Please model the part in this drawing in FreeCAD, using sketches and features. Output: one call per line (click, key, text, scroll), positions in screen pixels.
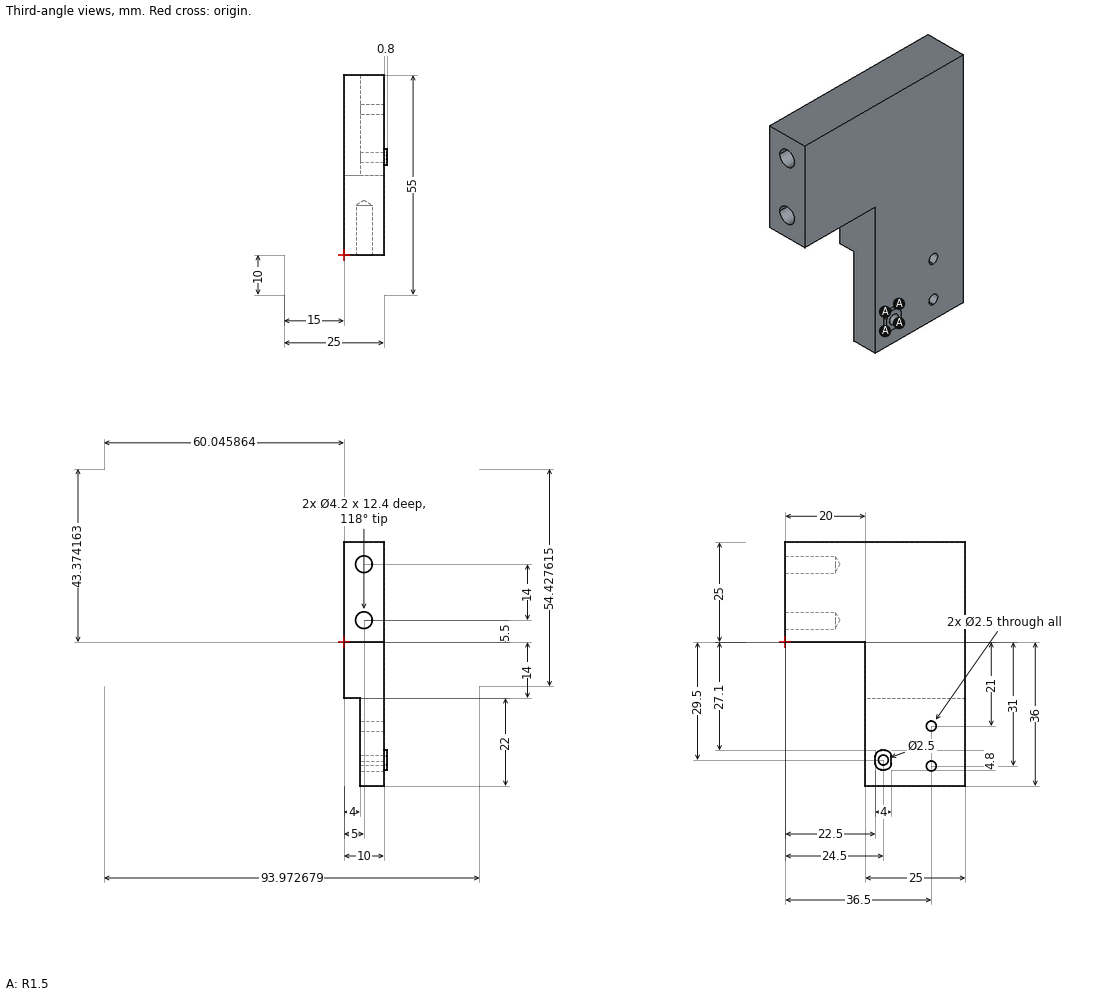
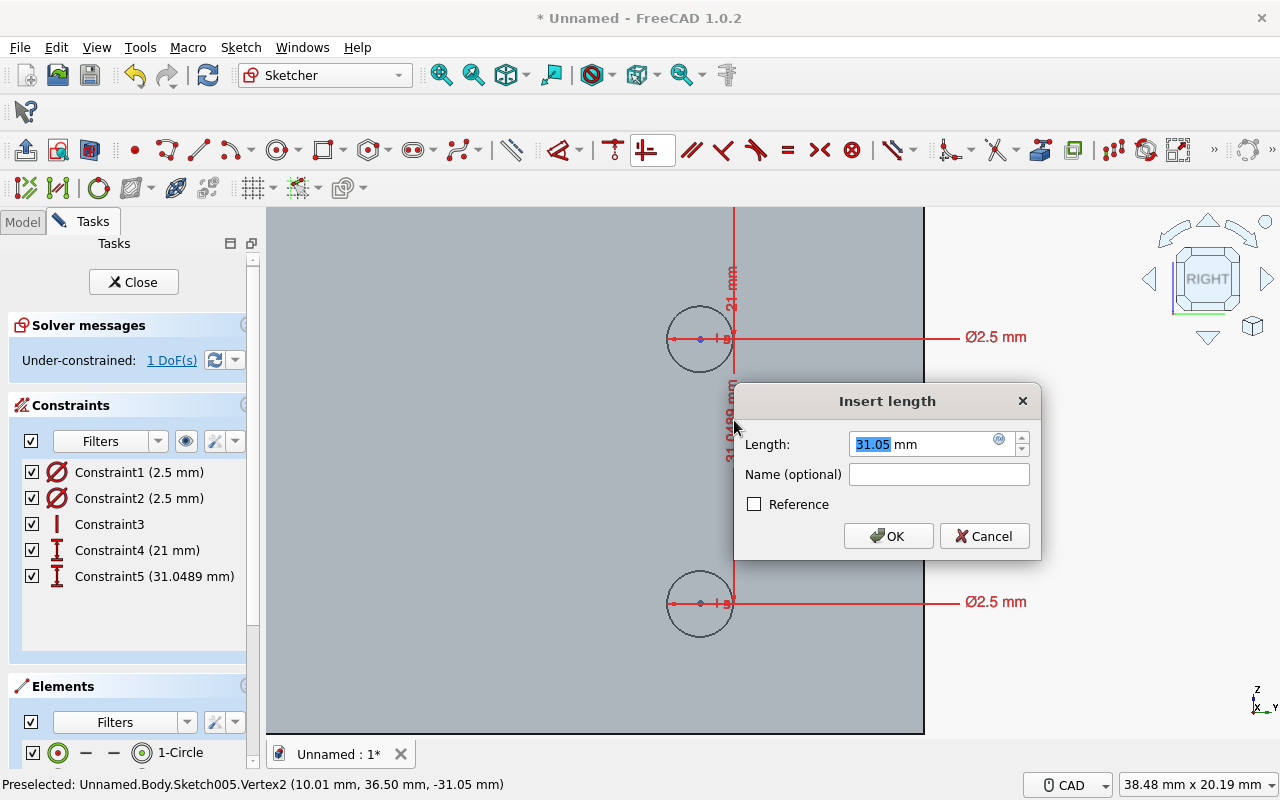
text(31)
key(Return)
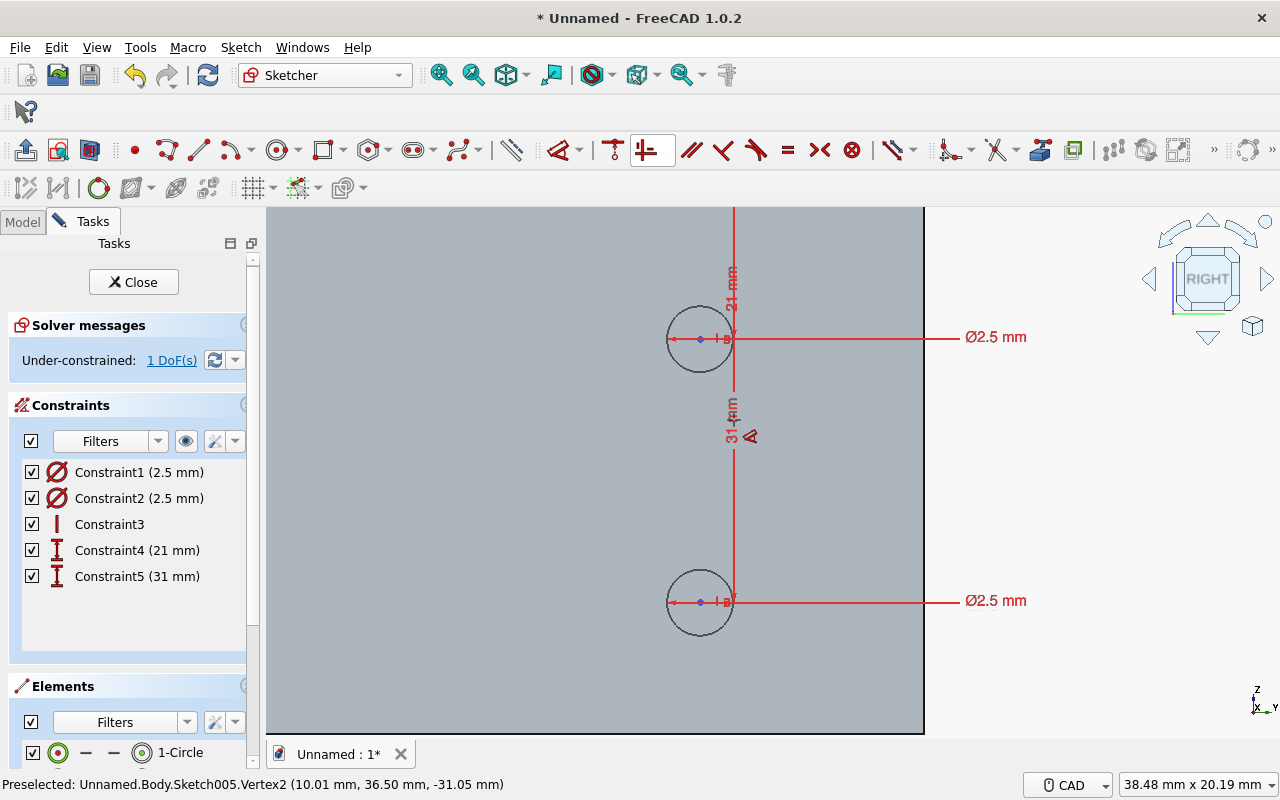
click(700, 339)
click(497, 373)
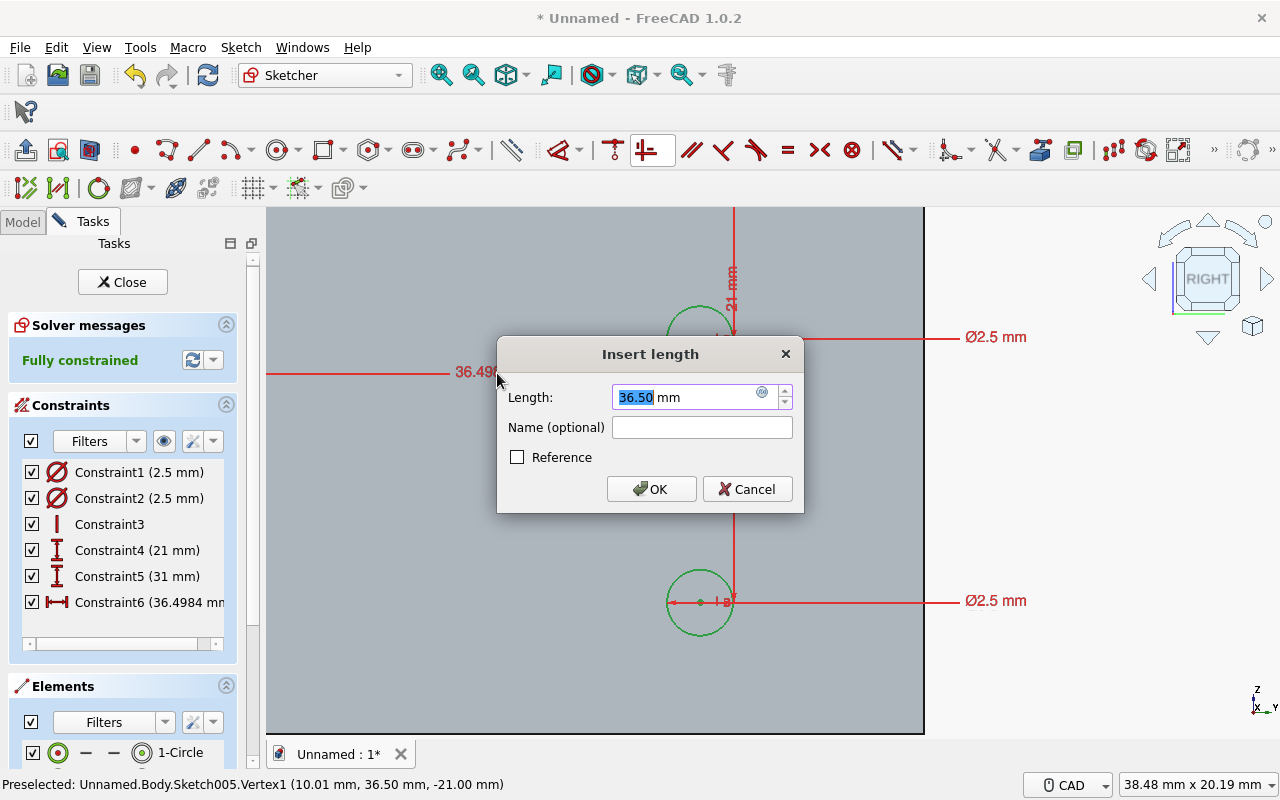
text(36.5)
key(Return)
key(Escape)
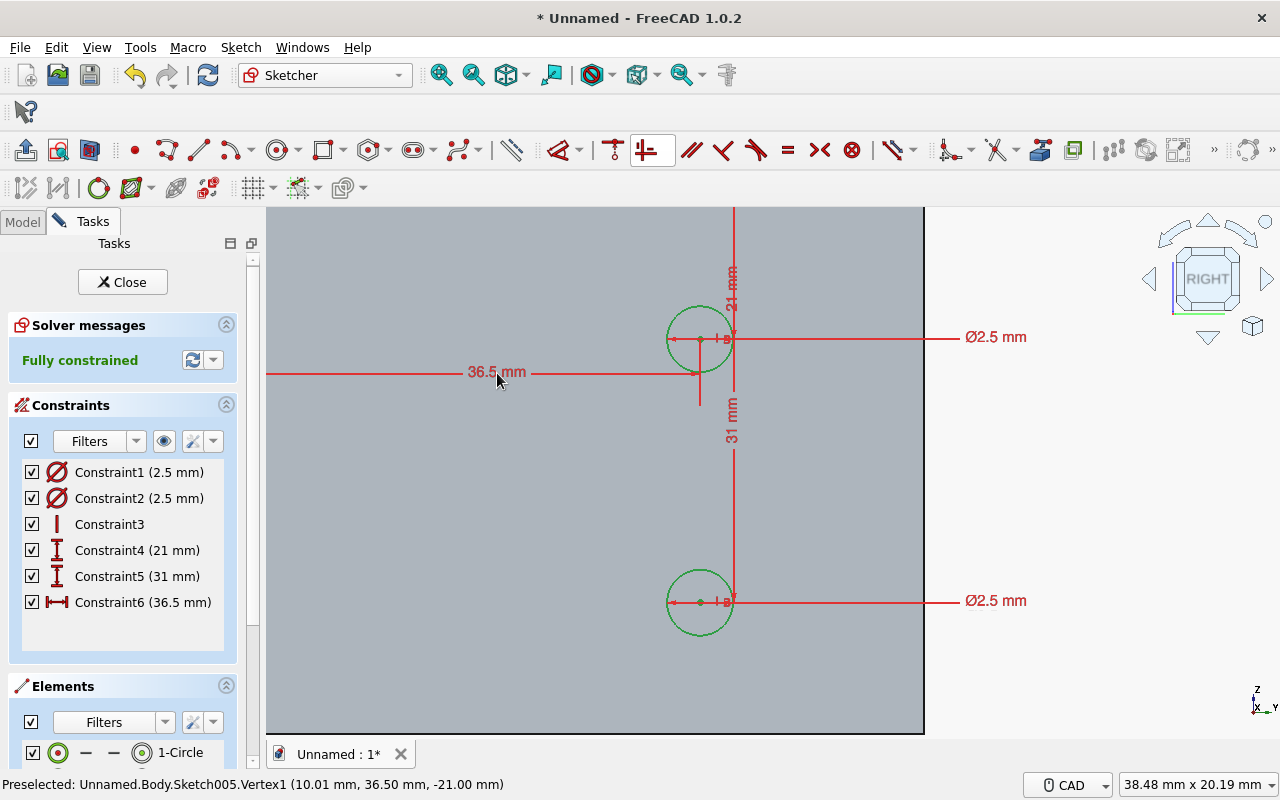
click(123, 282)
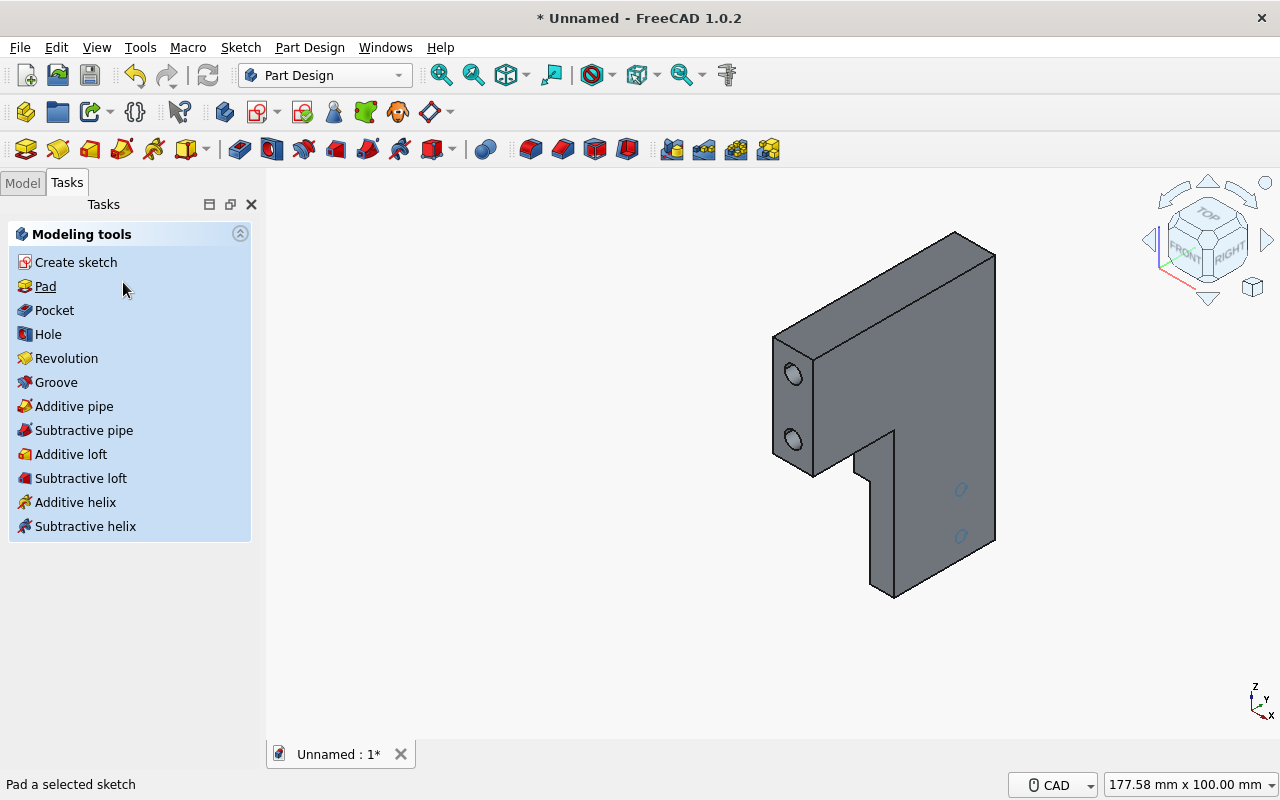
click(272, 150)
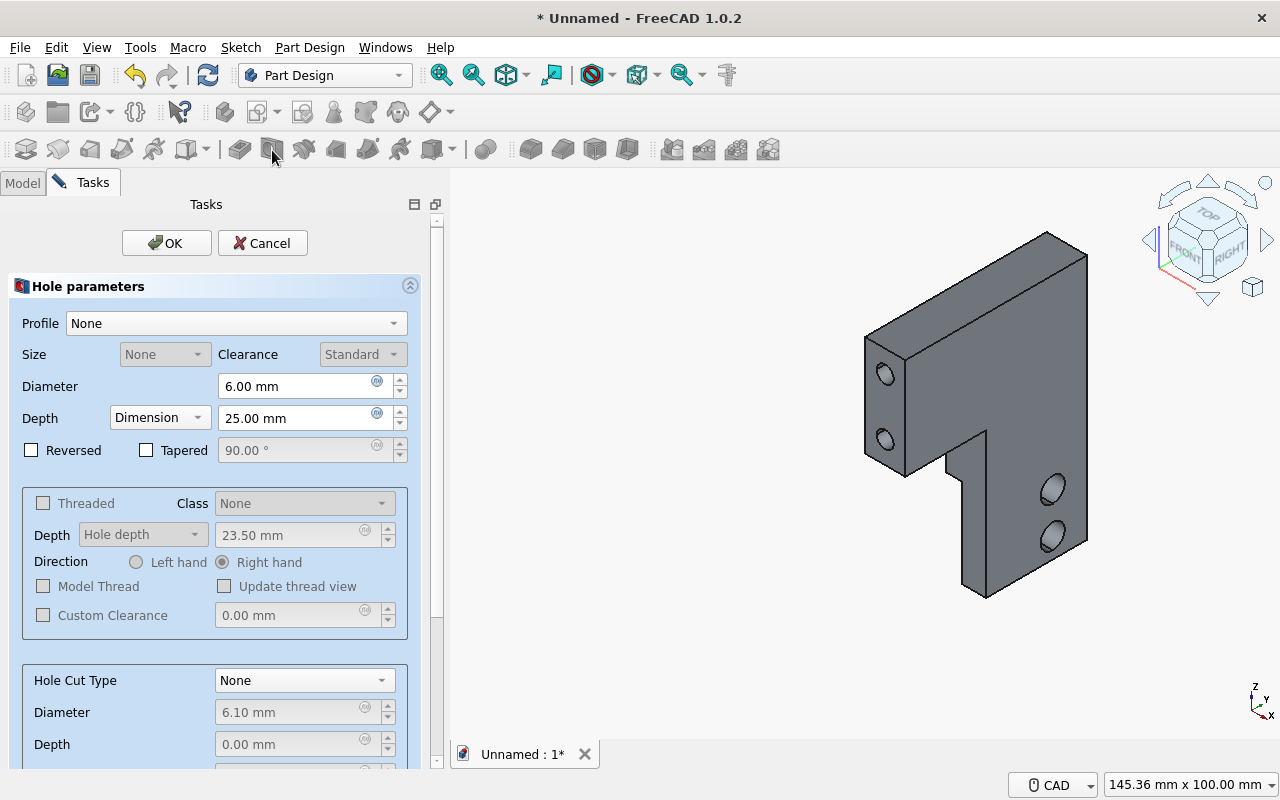
triple_click(305, 386)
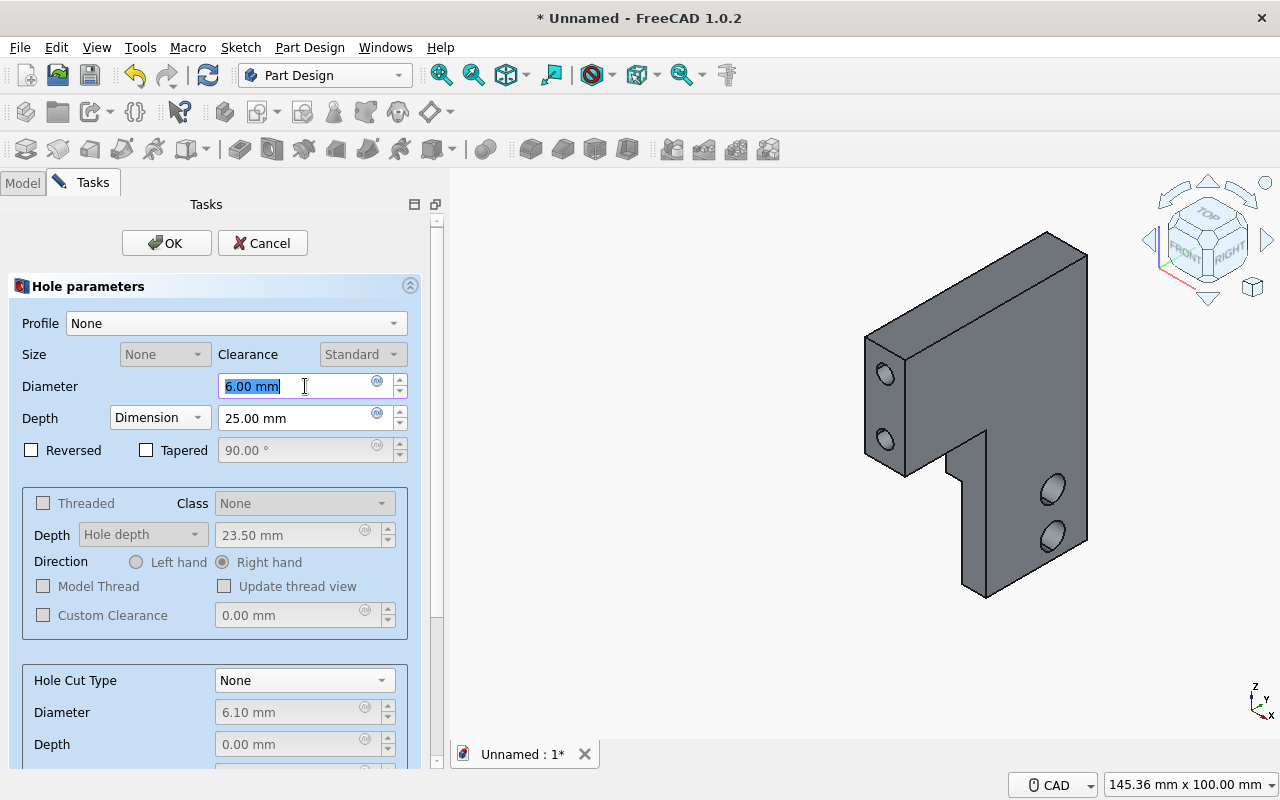
text(2.5)
key(Tab)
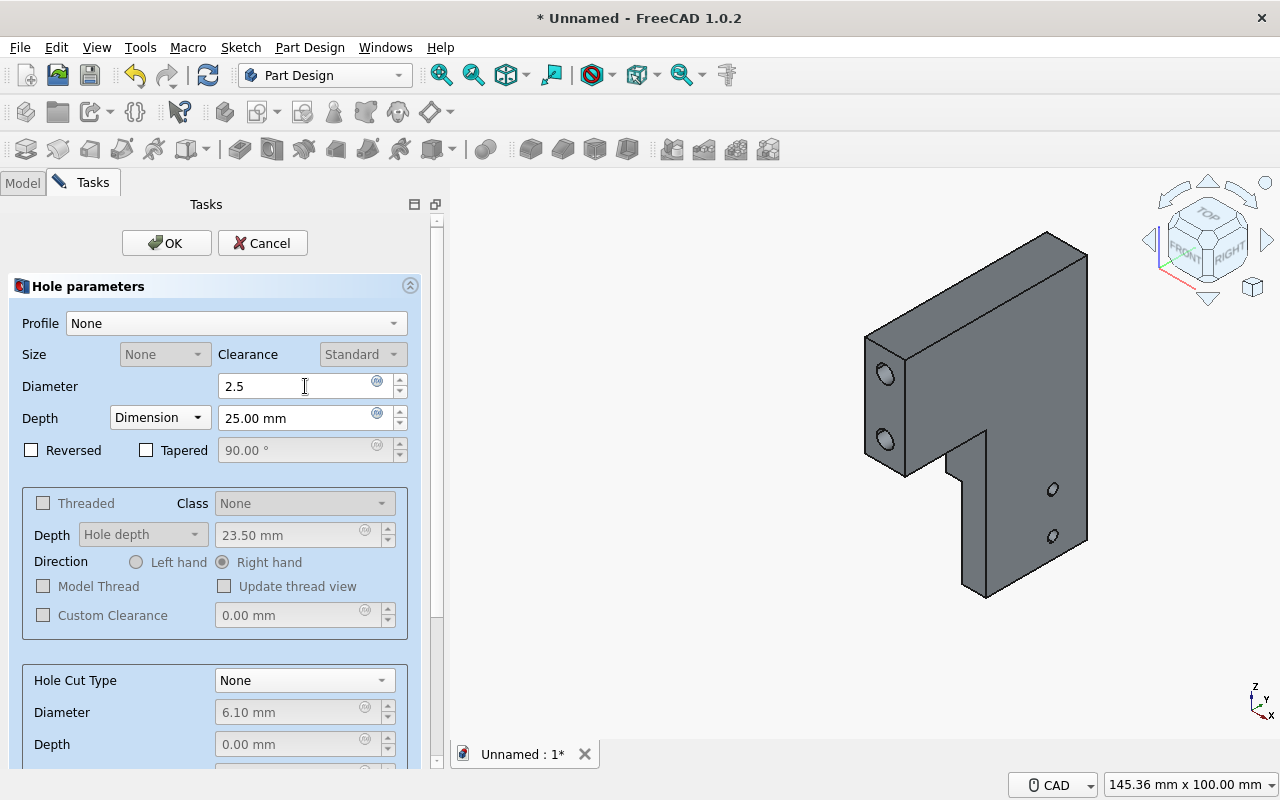
click(161, 418)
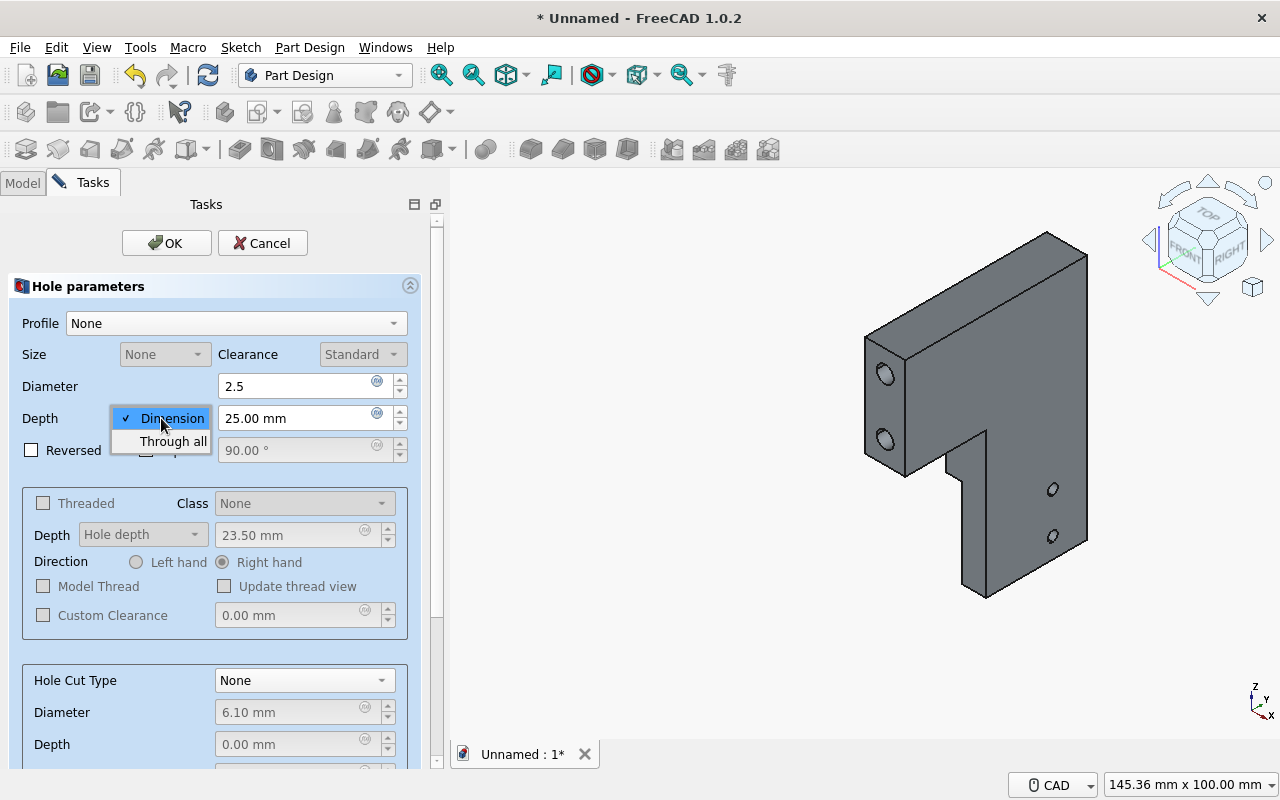
click(160, 442)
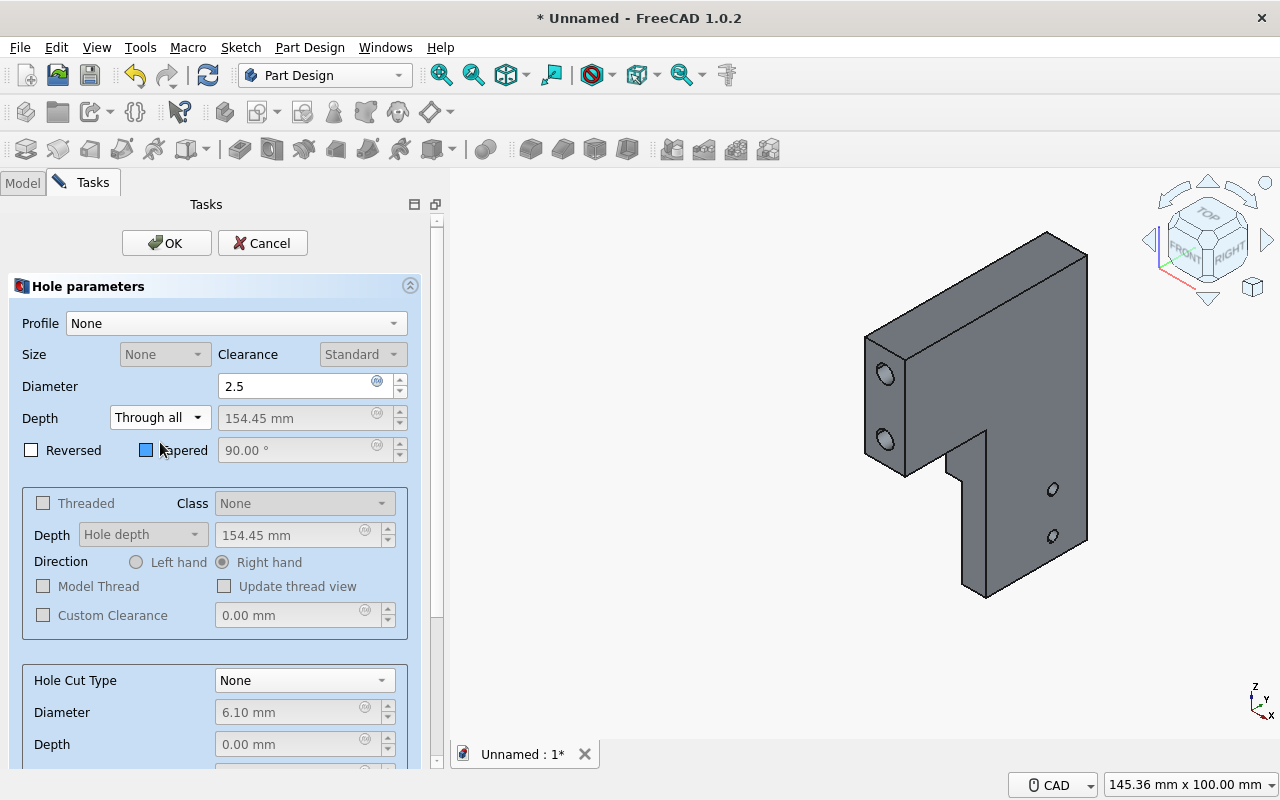
click(167, 243)